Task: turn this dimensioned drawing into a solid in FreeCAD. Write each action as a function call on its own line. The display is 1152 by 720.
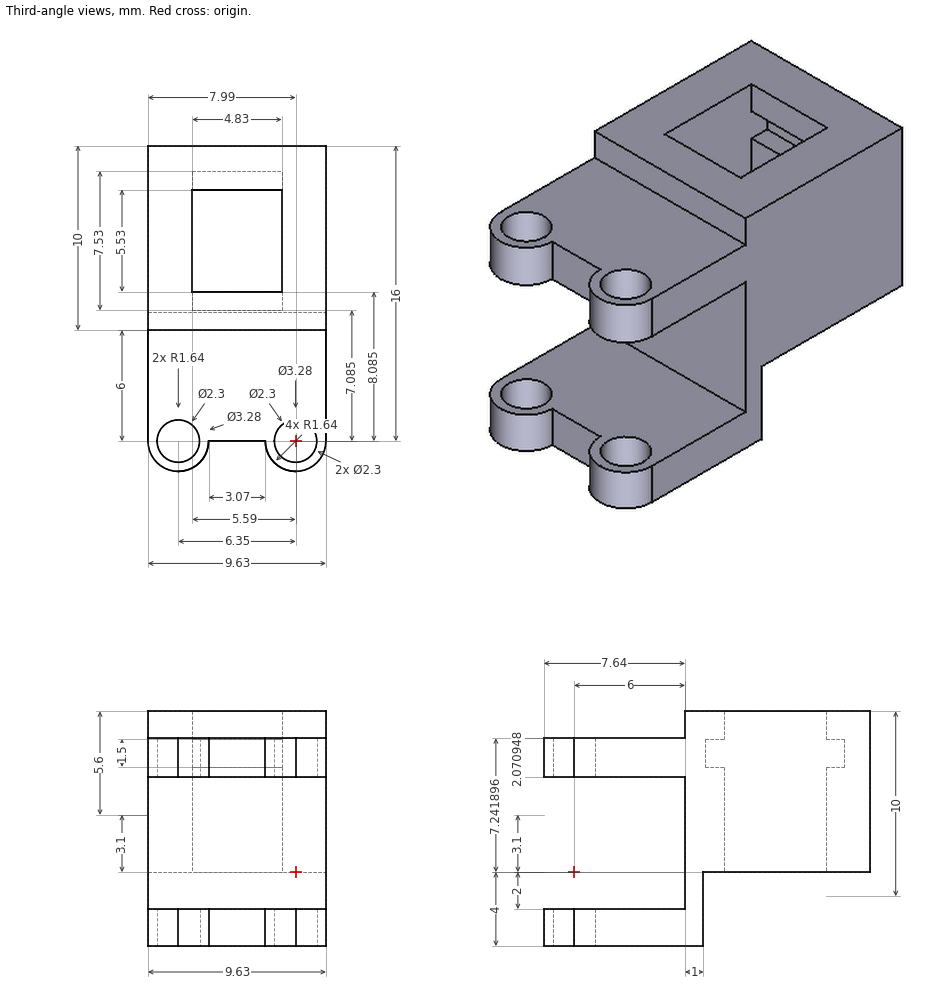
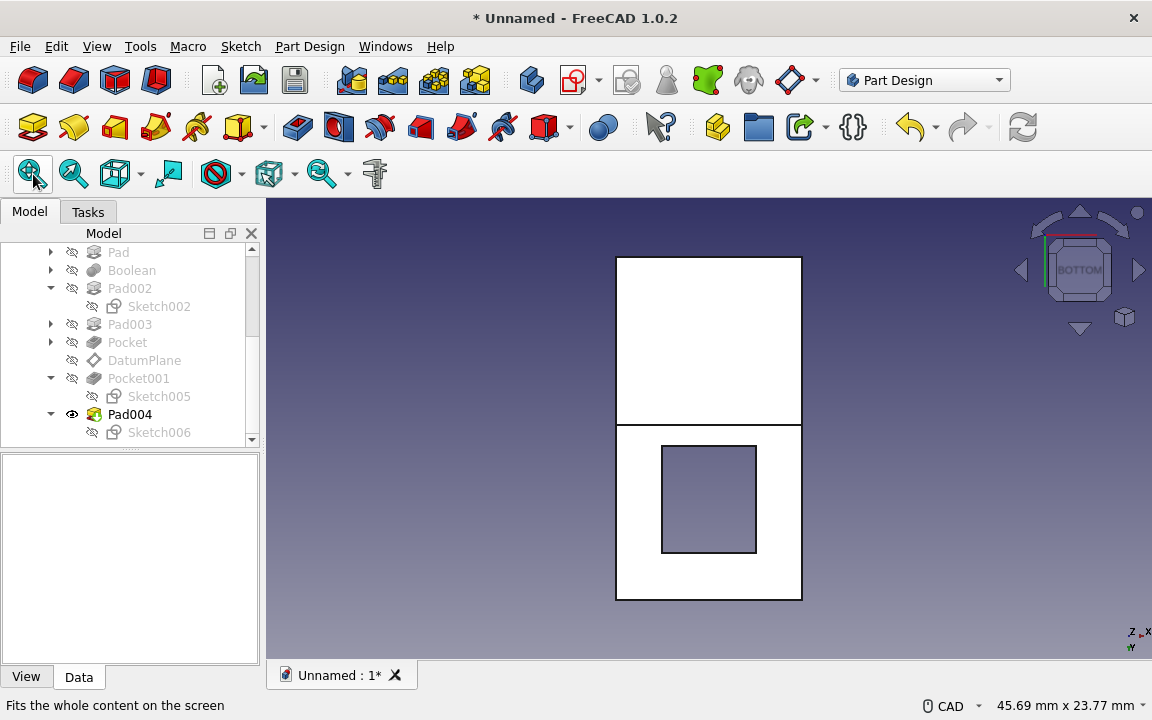
click(709, 340)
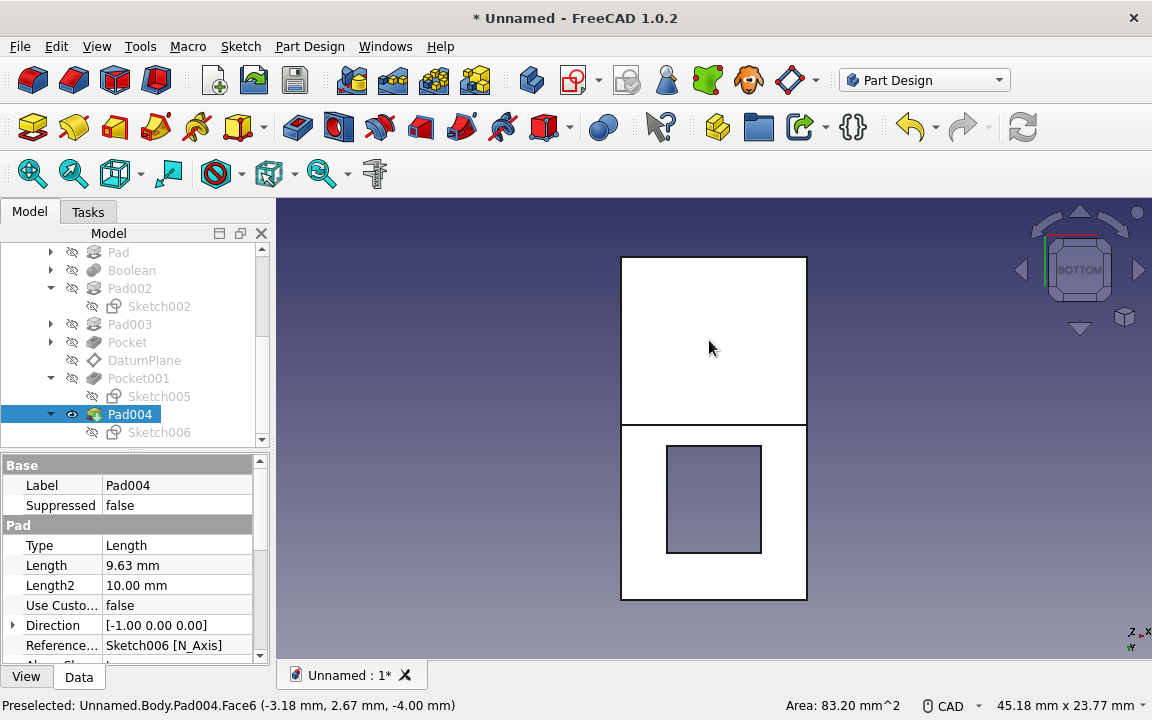
click(572, 80)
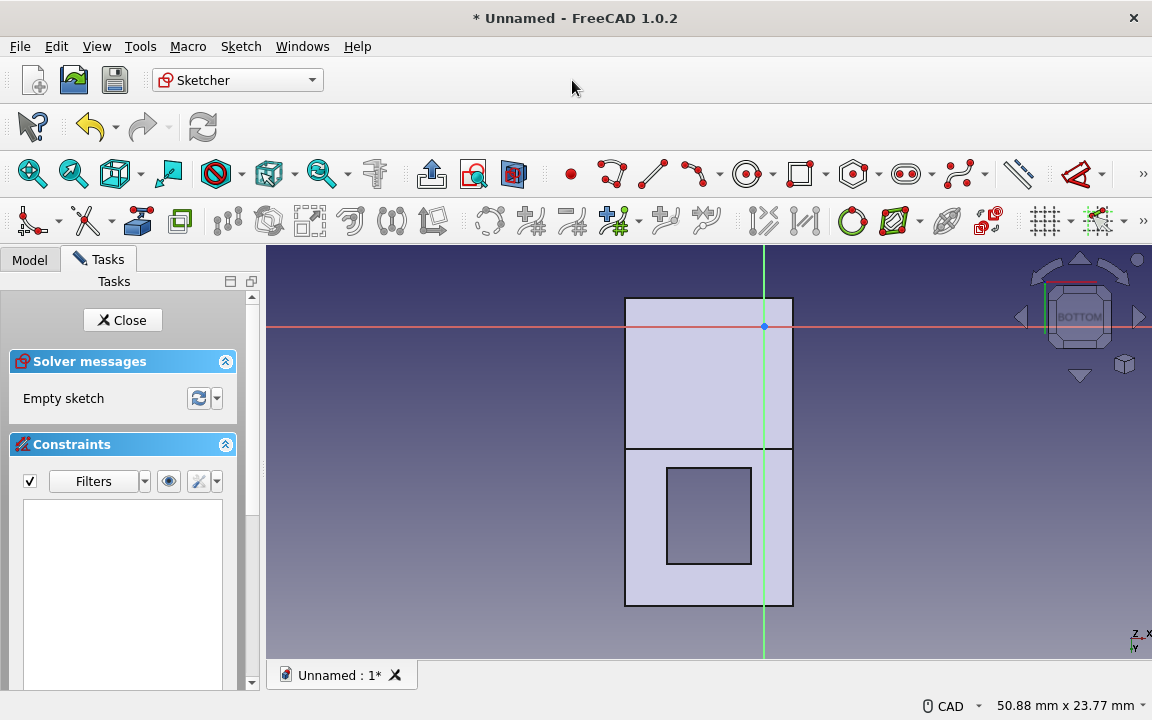
scroll(739, 273, up, 6)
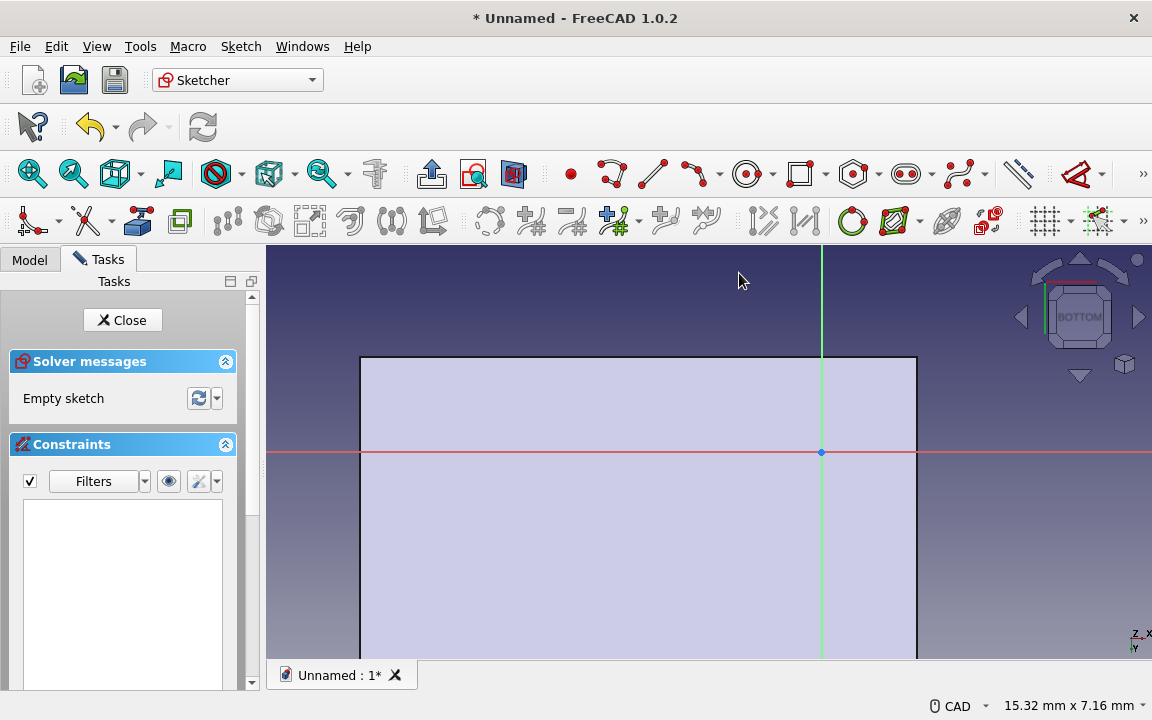
click(746, 174)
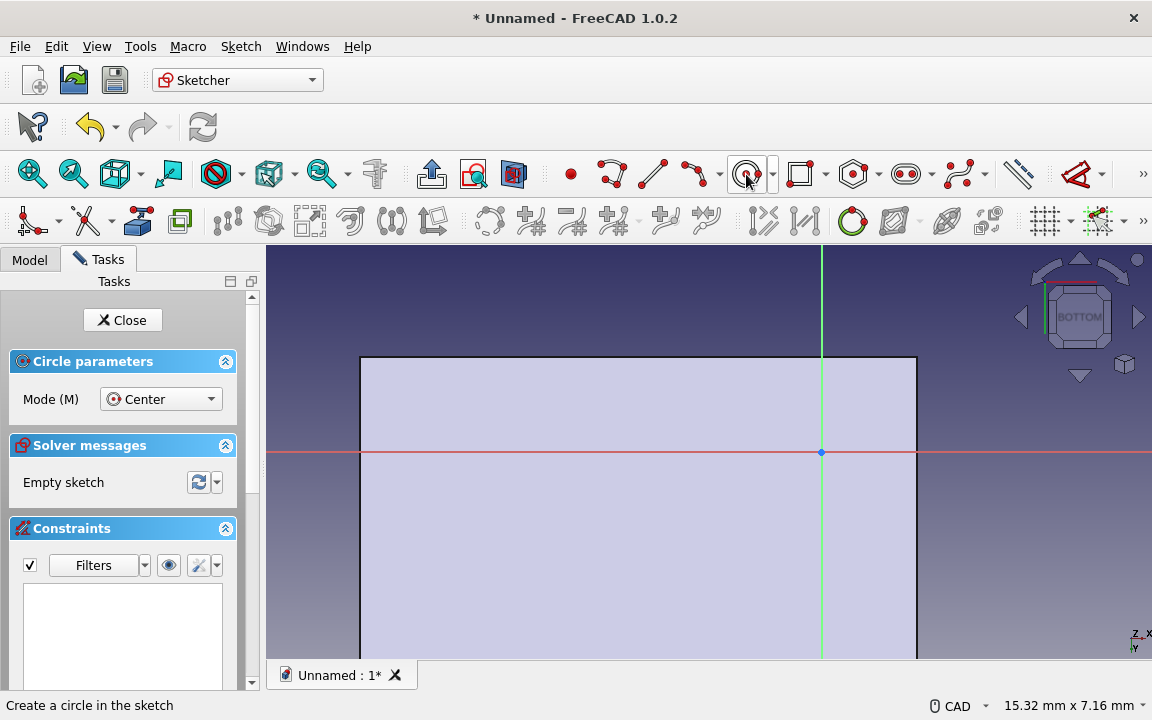
click(822, 452)
click(869, 405)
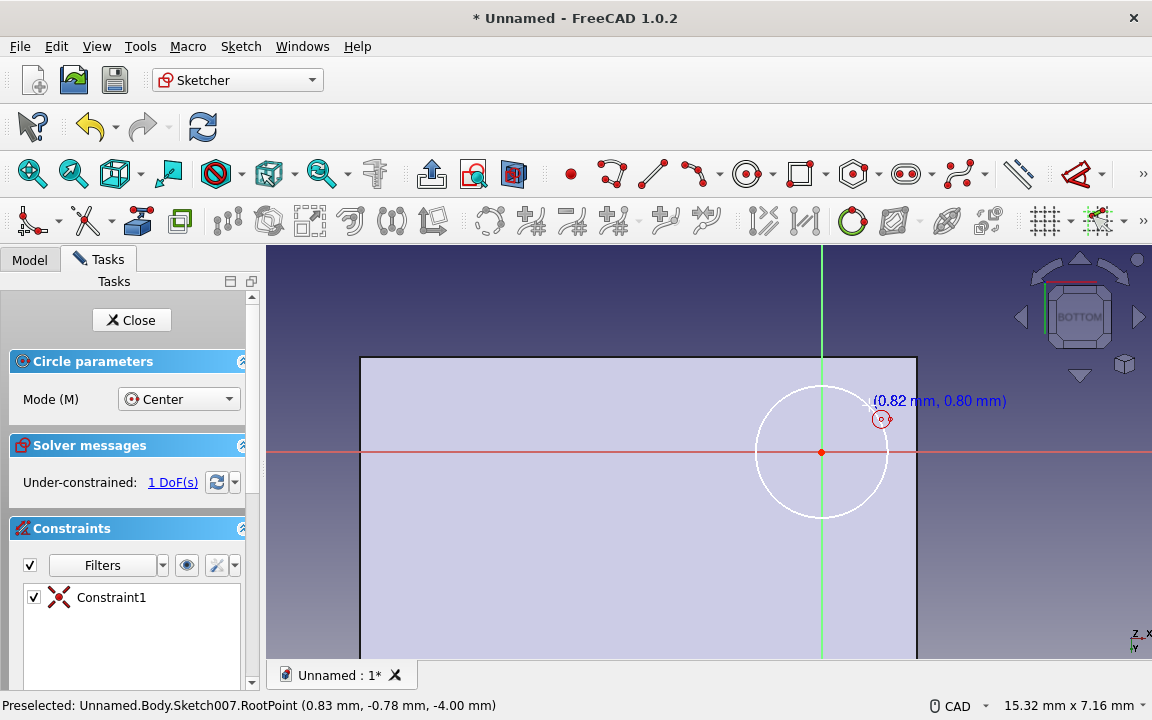
click(455, 452)
click(502, 405)
key(Escape)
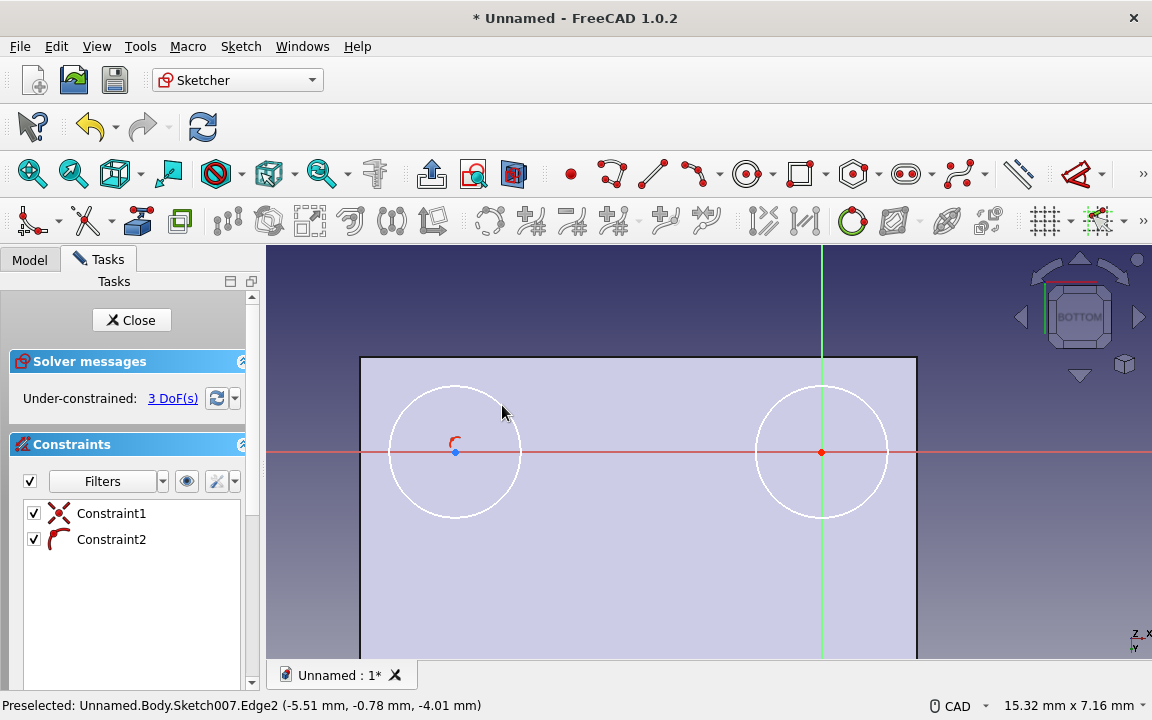
click(868, 405)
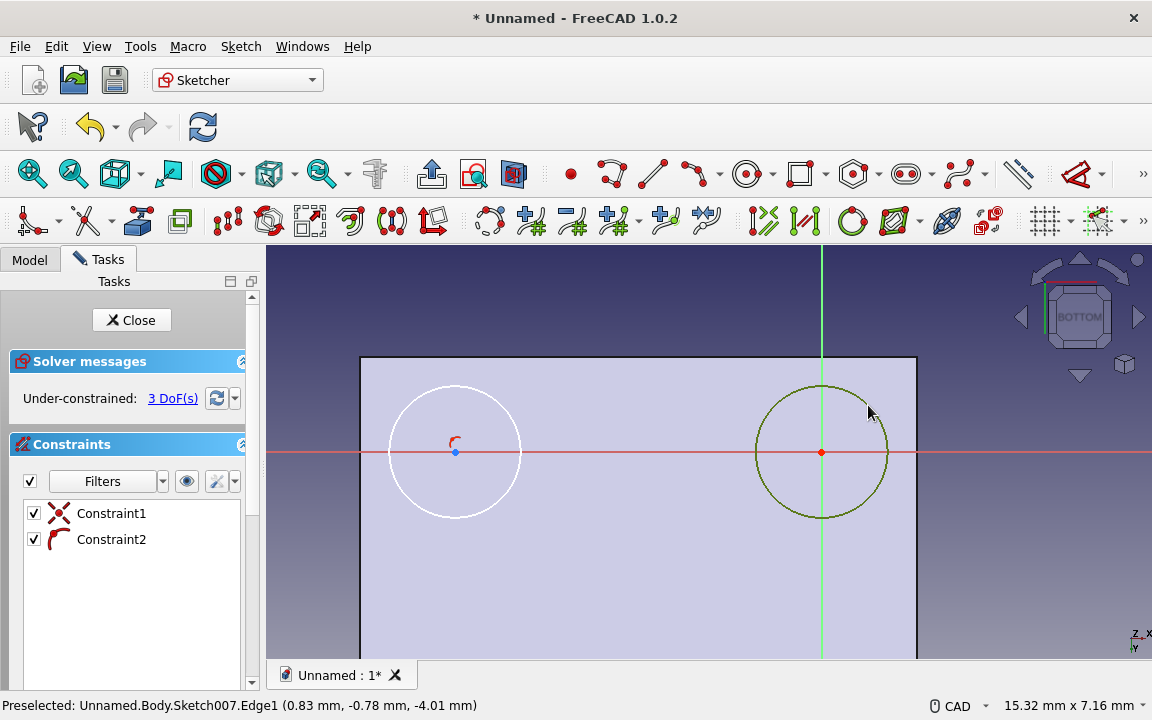
click(501, 405)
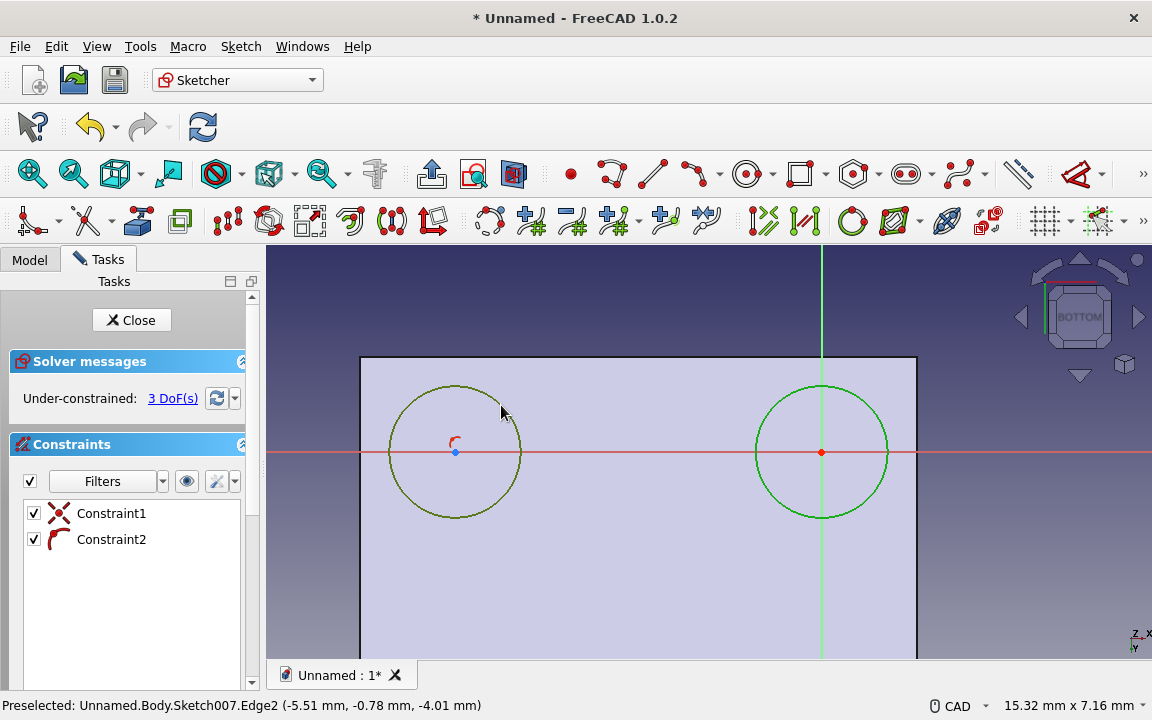
key(e)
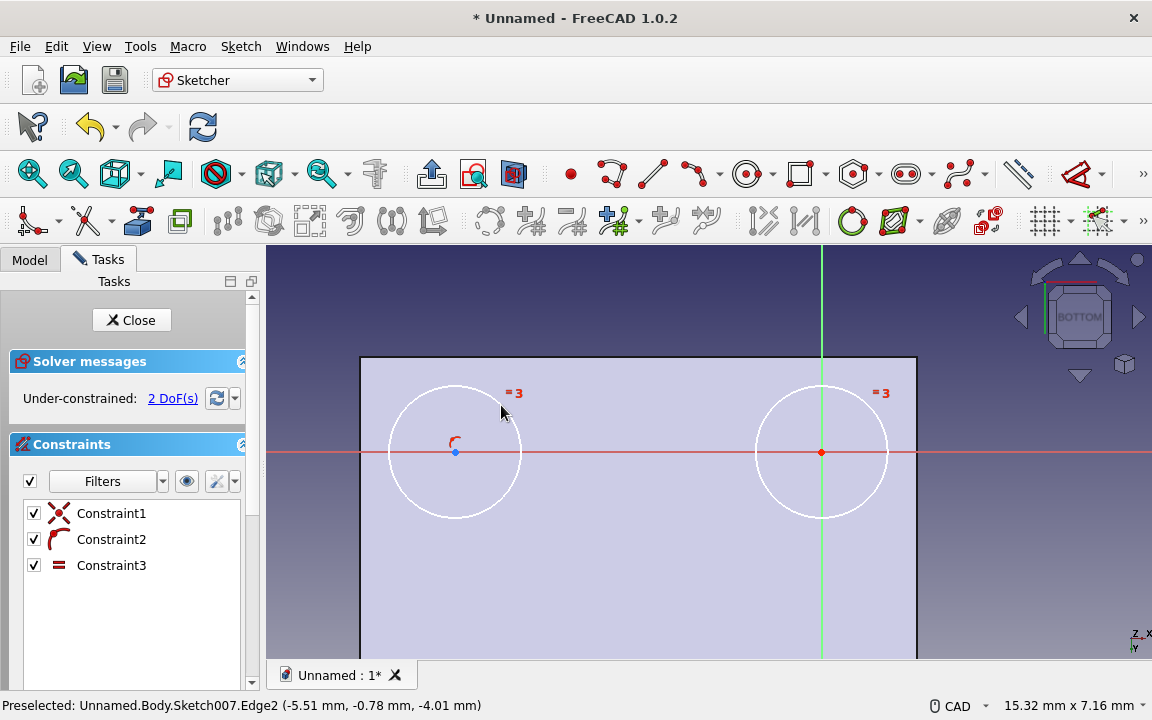
click(1076, 174)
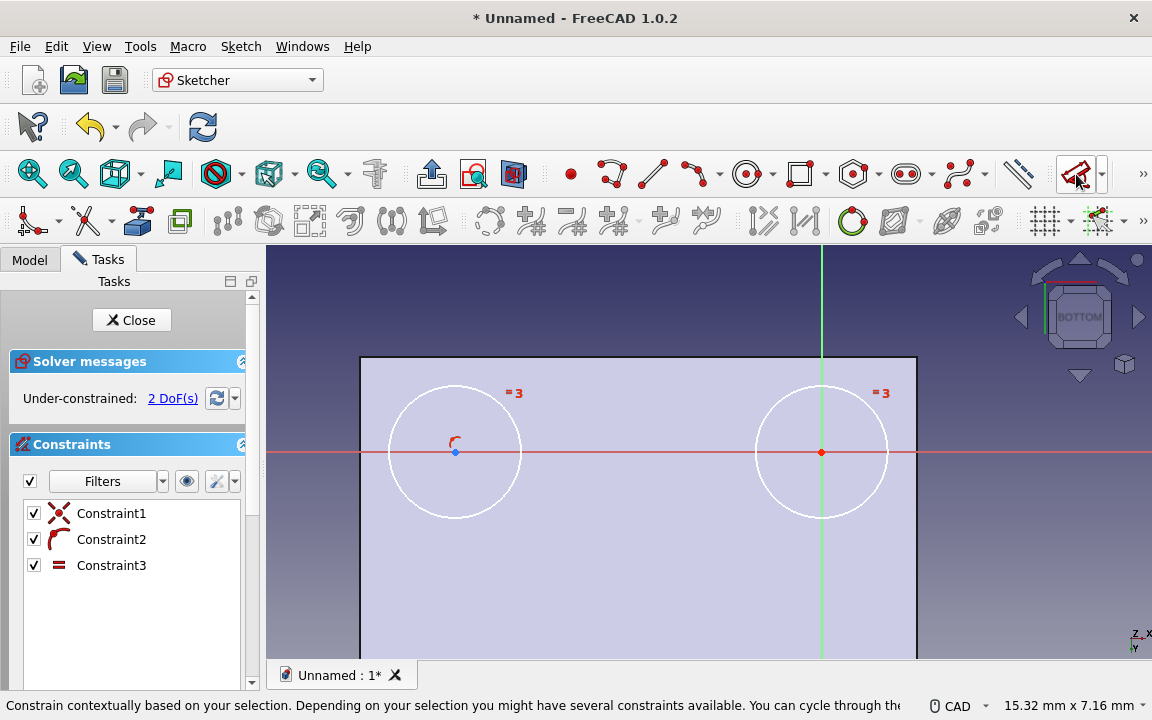
click(868, 405)
click(890, 382)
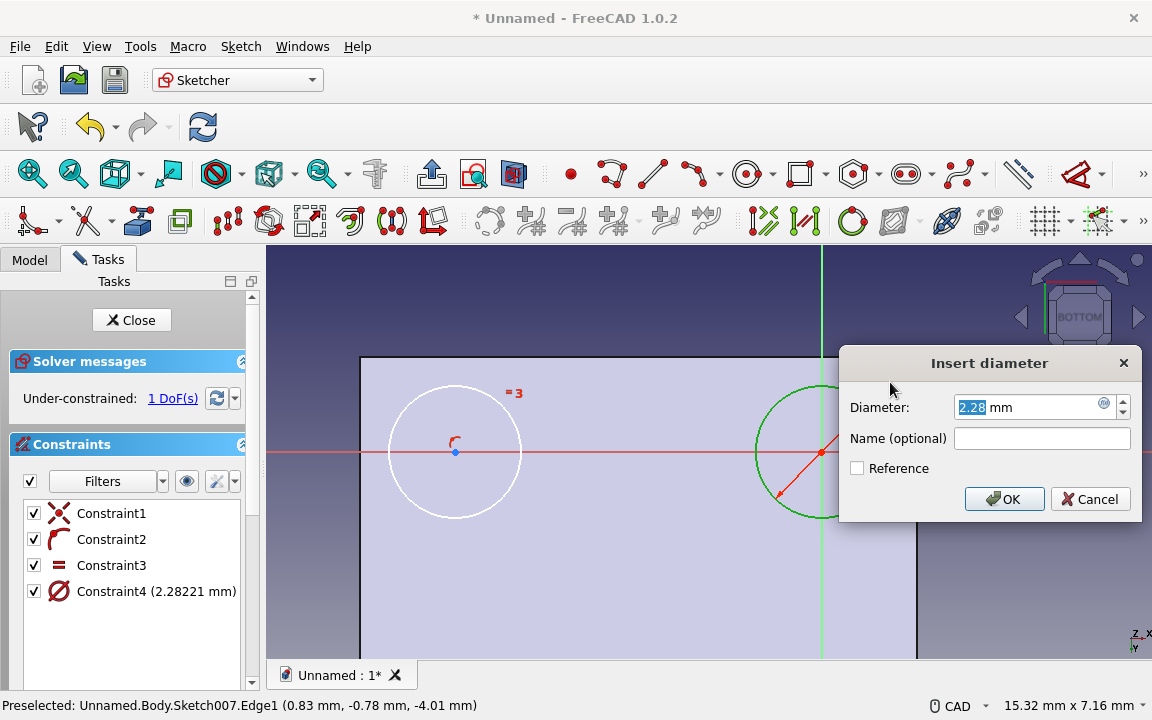
text(2.3)
key(Return)